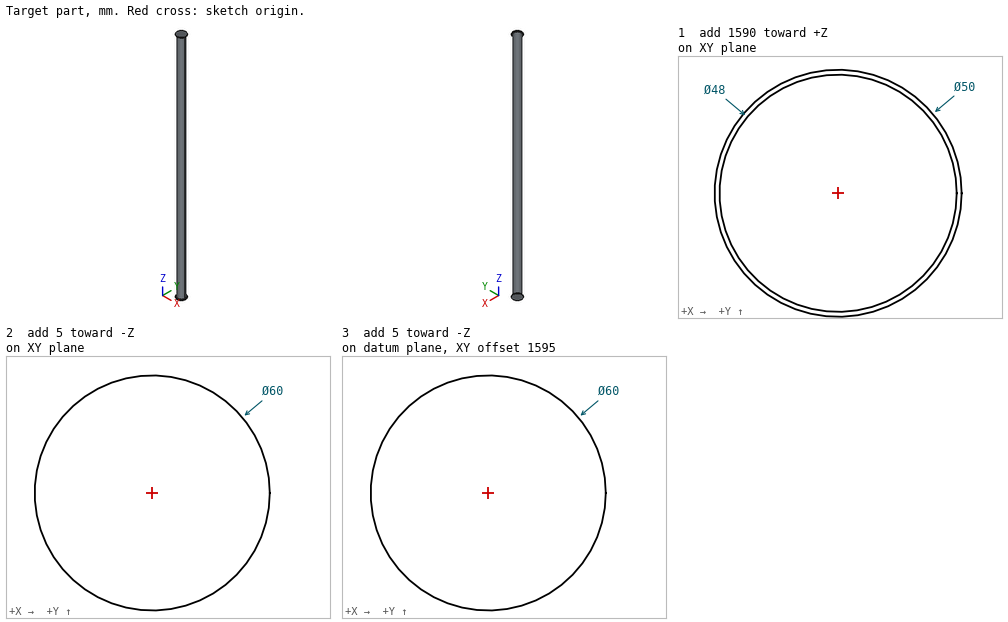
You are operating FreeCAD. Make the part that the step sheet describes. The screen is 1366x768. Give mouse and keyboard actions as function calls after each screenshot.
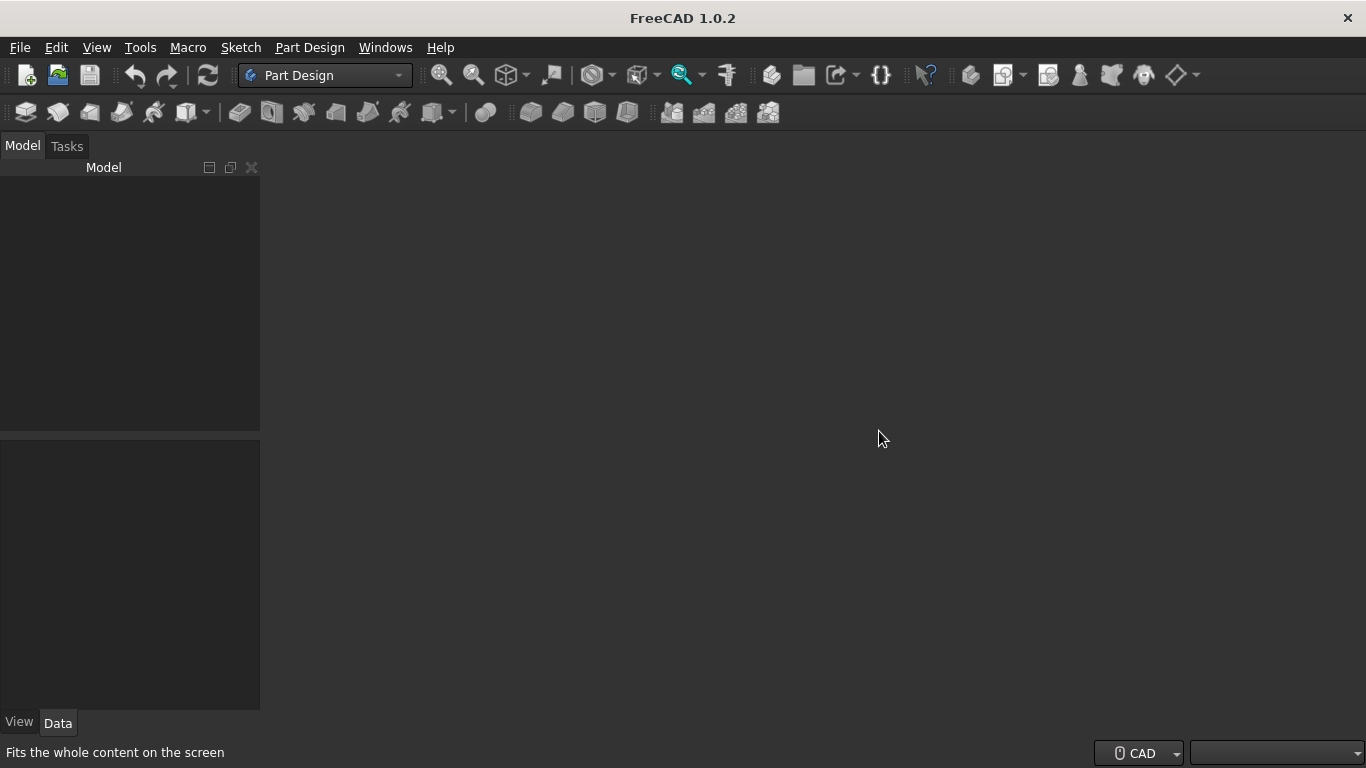
click(26, 76)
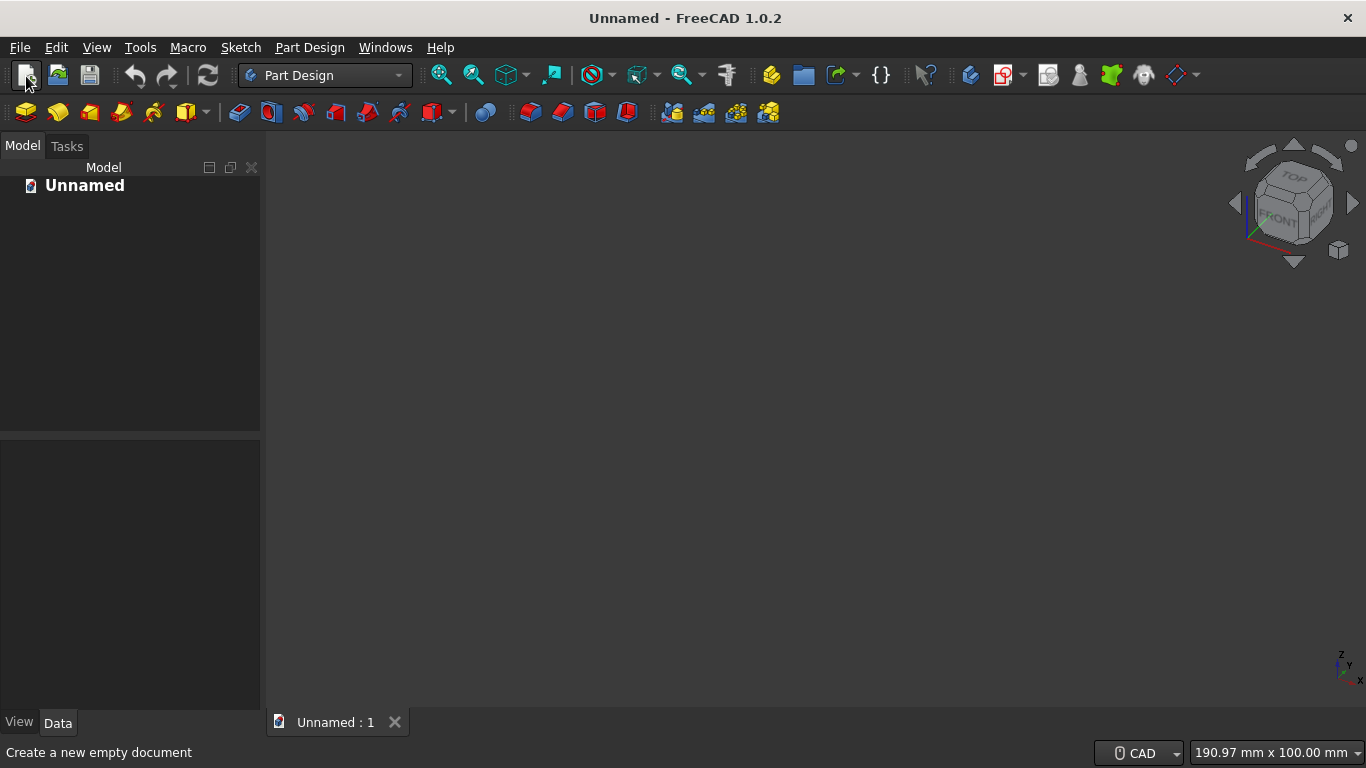
click(1004, 76)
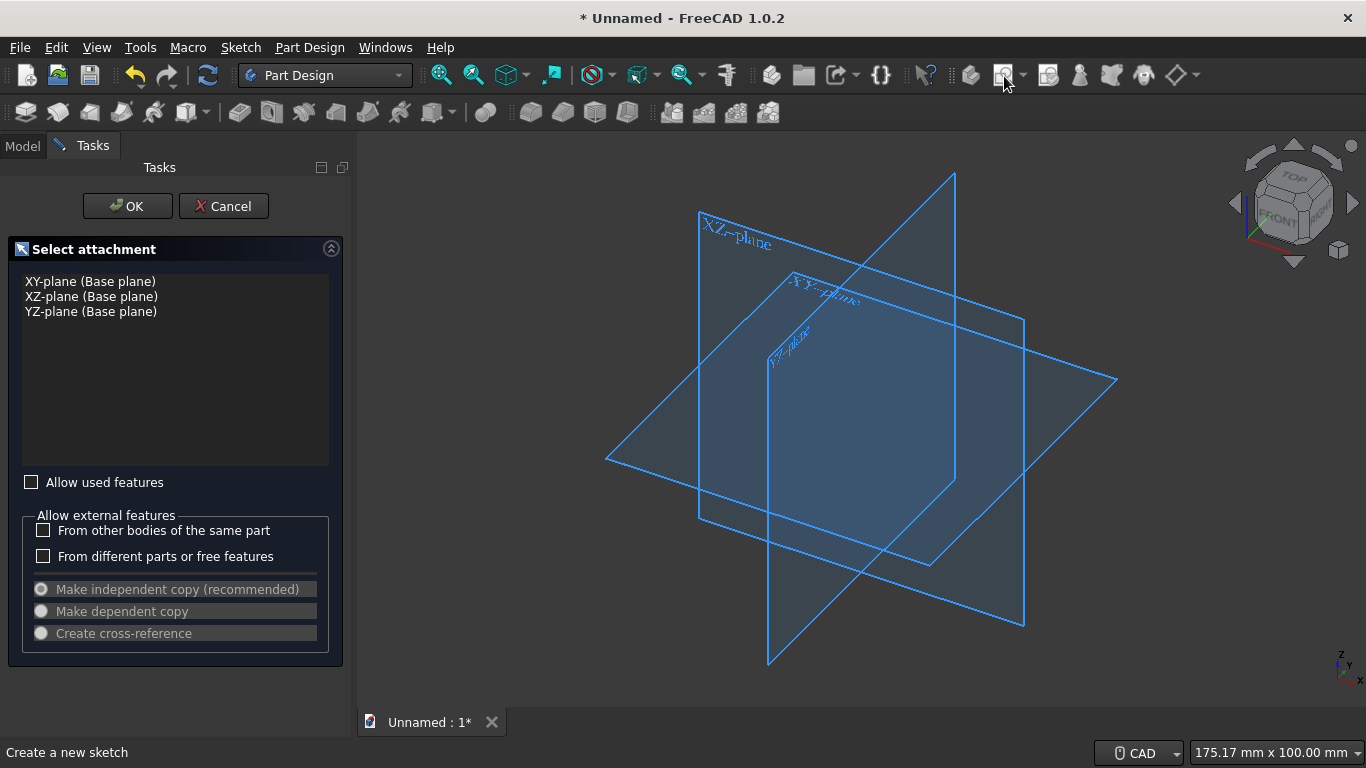
click(82, 282)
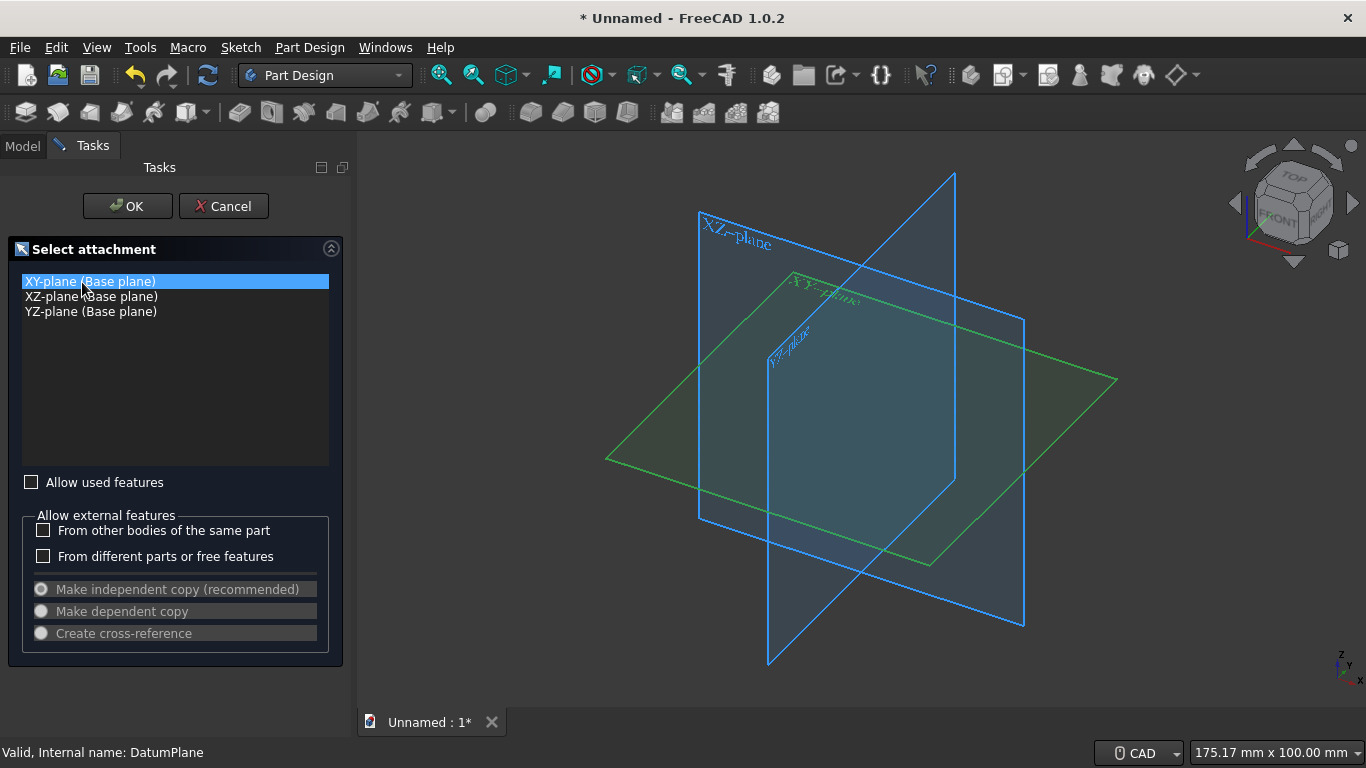
click(128, 206)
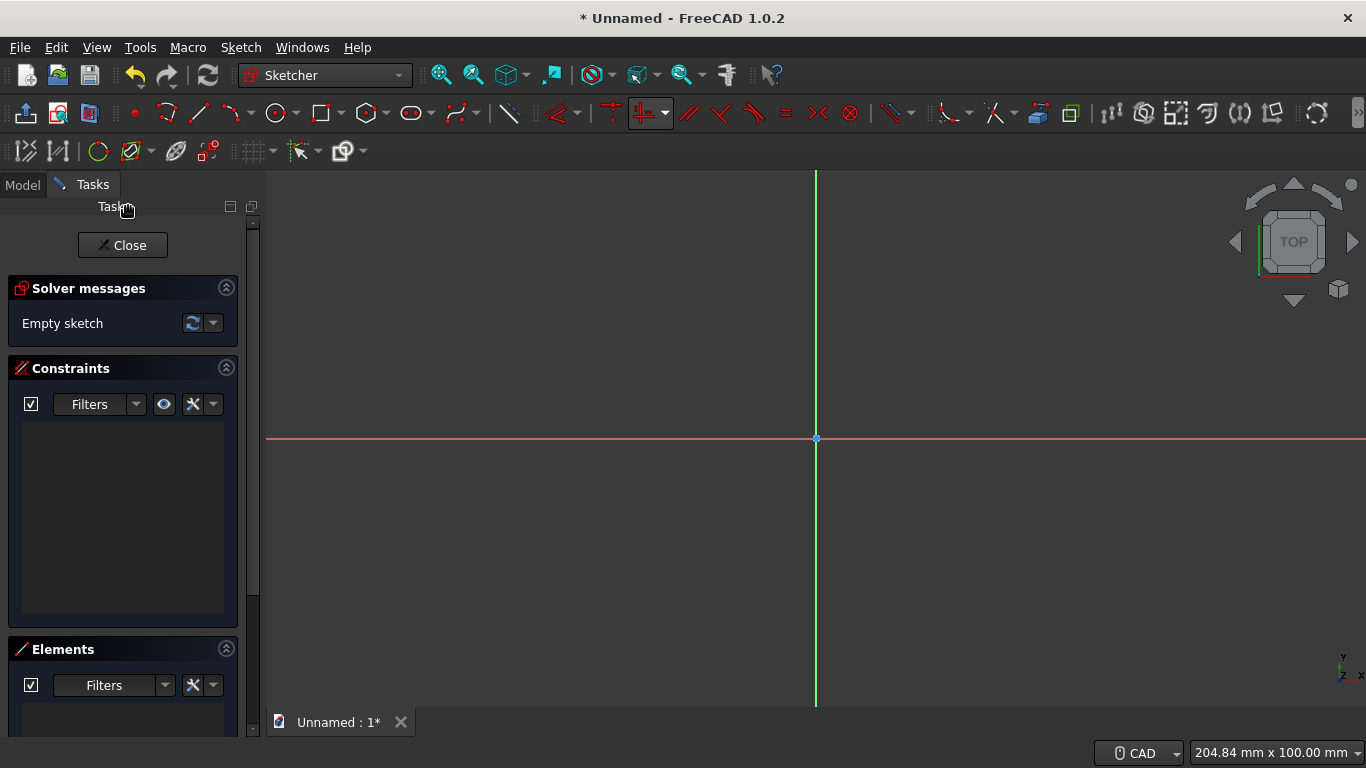
click(276, 114)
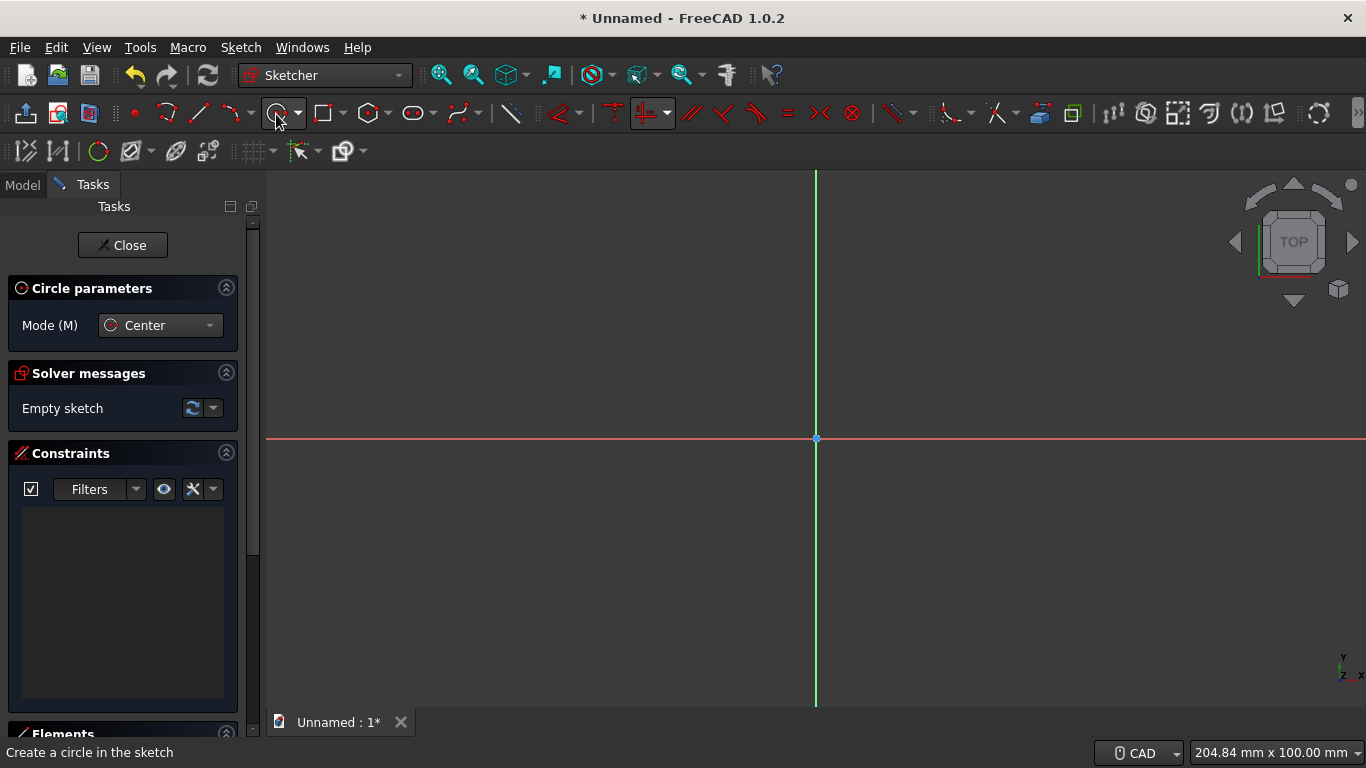
click(816, 438)
move(911, 344)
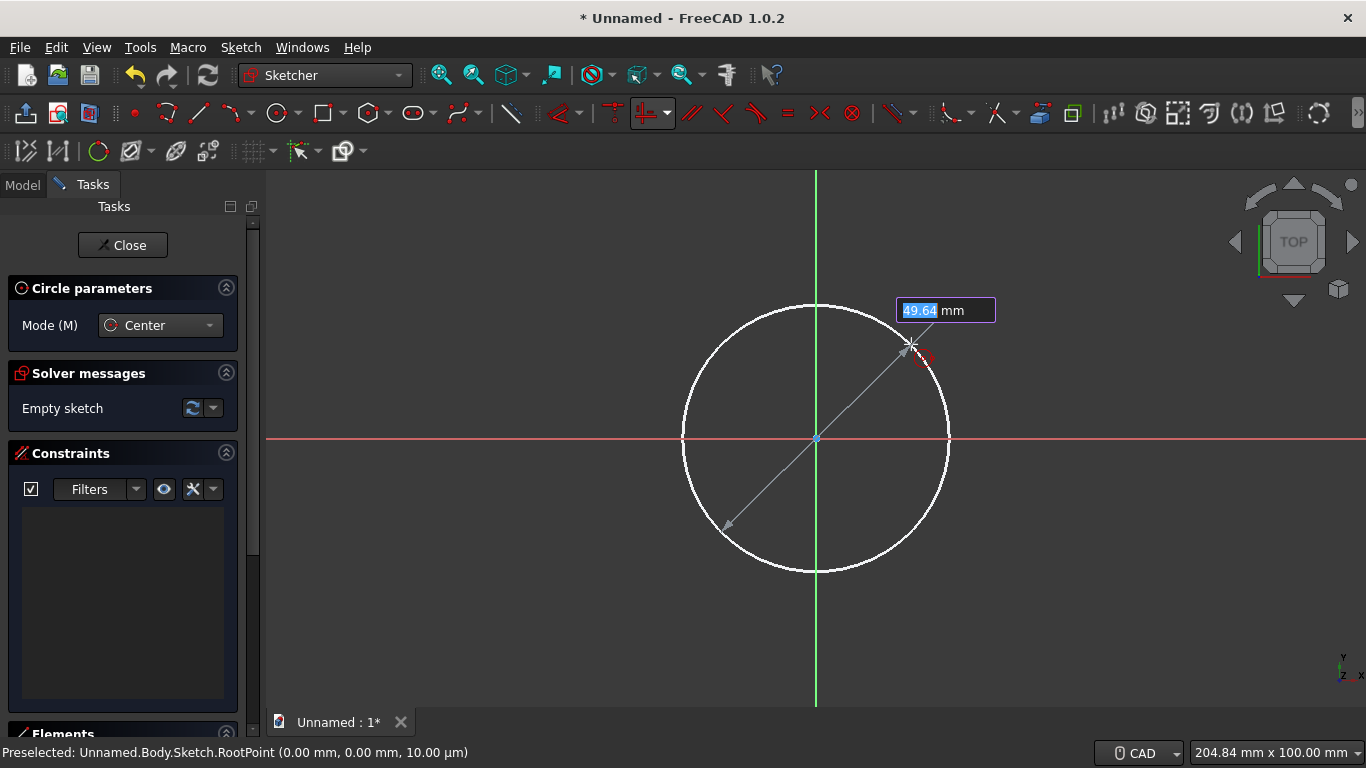
text(50)
key(Return)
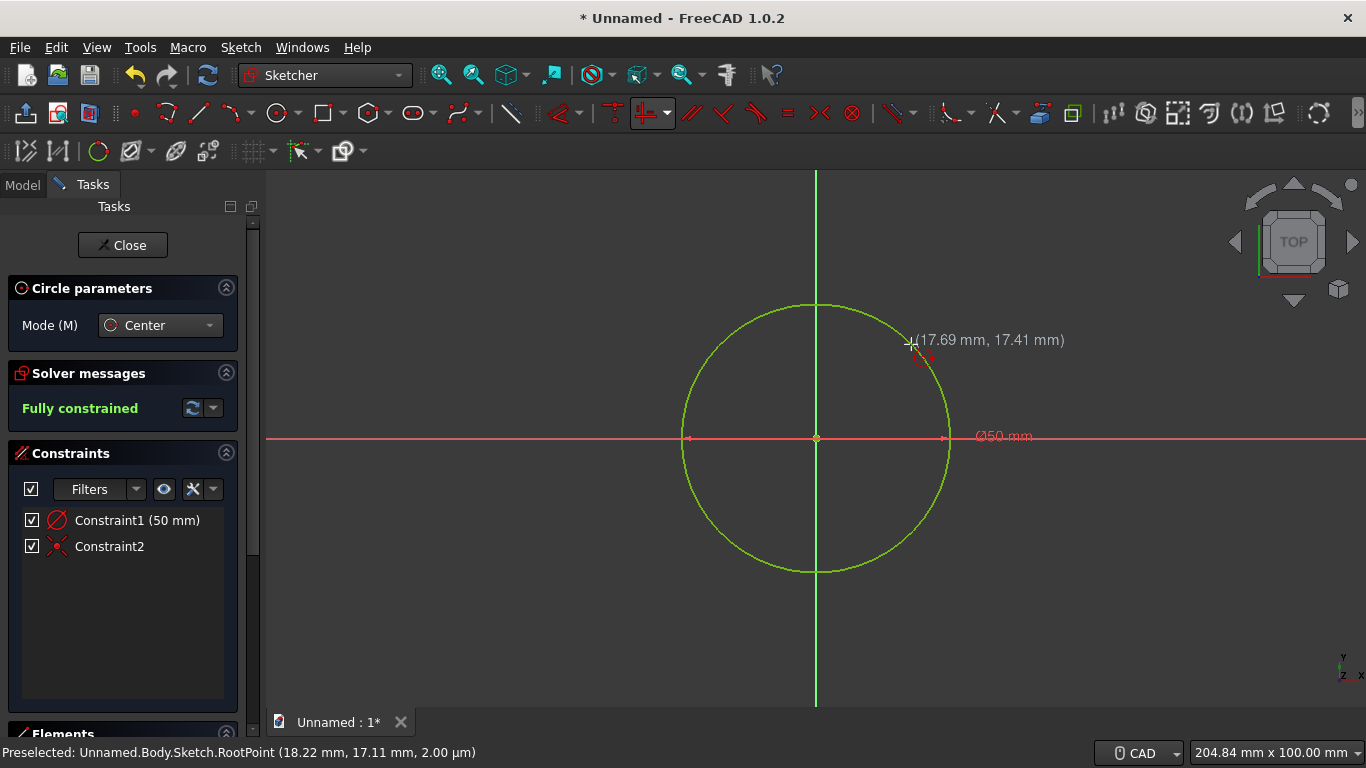
click(816, 438)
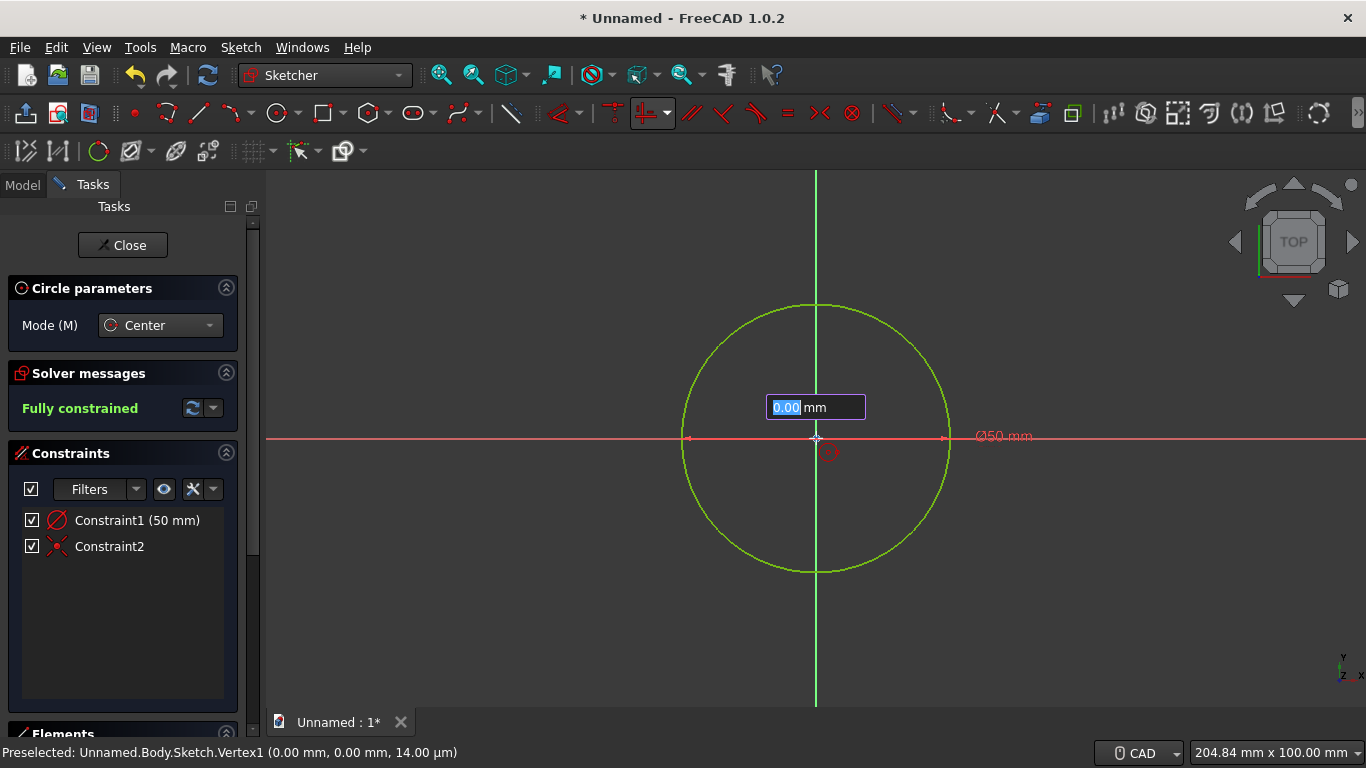
scroll(907, 530, up, 6)
move(906, 527)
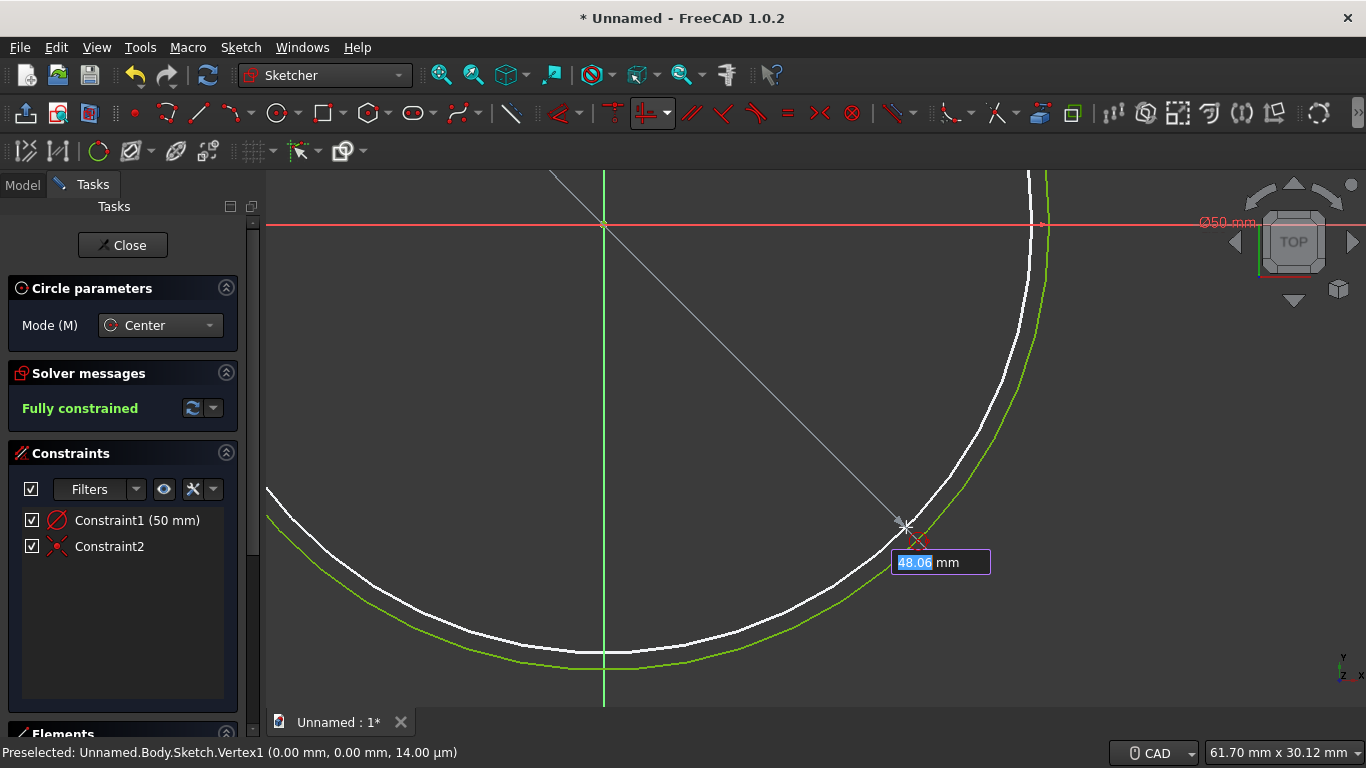
text(48)
key(Return)
key(Escape)